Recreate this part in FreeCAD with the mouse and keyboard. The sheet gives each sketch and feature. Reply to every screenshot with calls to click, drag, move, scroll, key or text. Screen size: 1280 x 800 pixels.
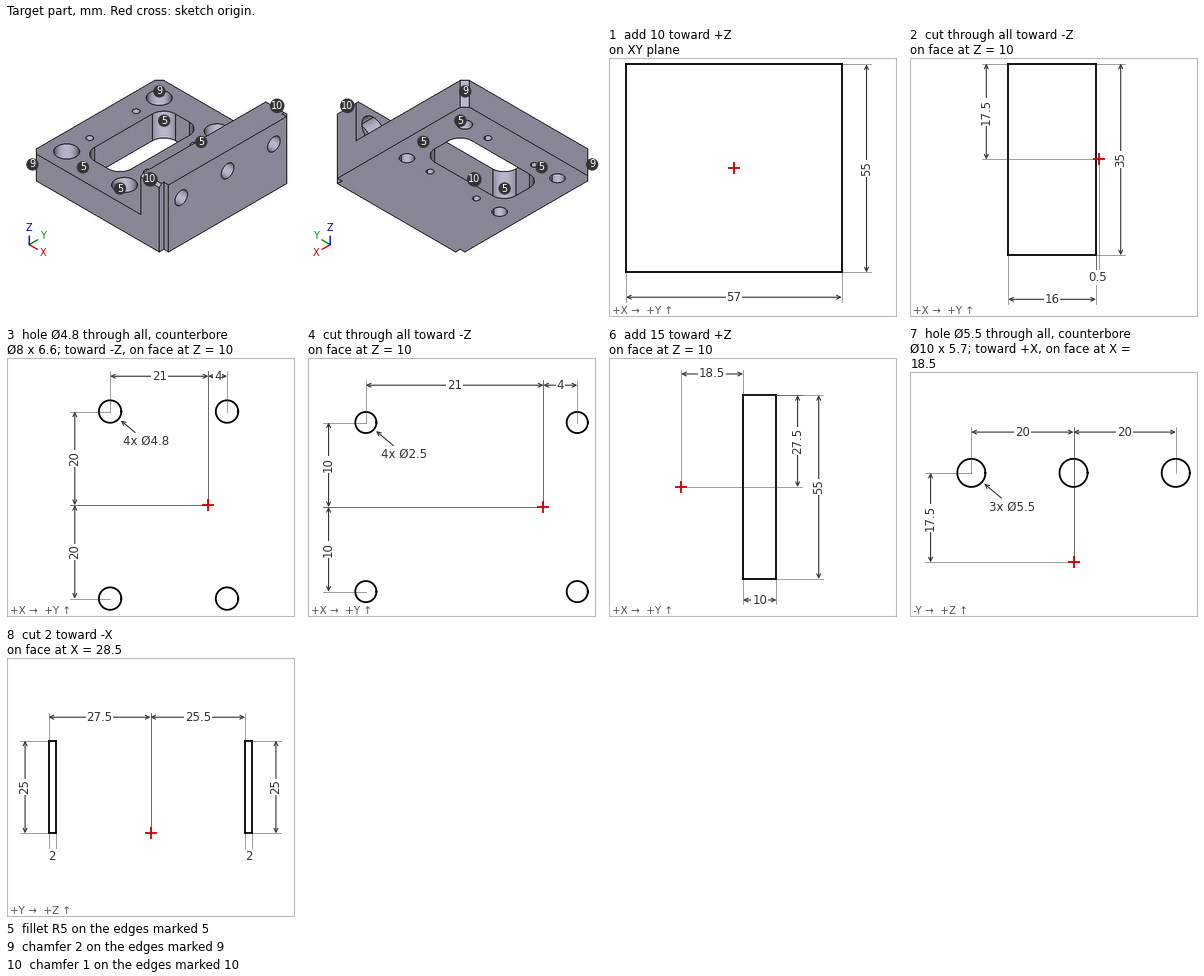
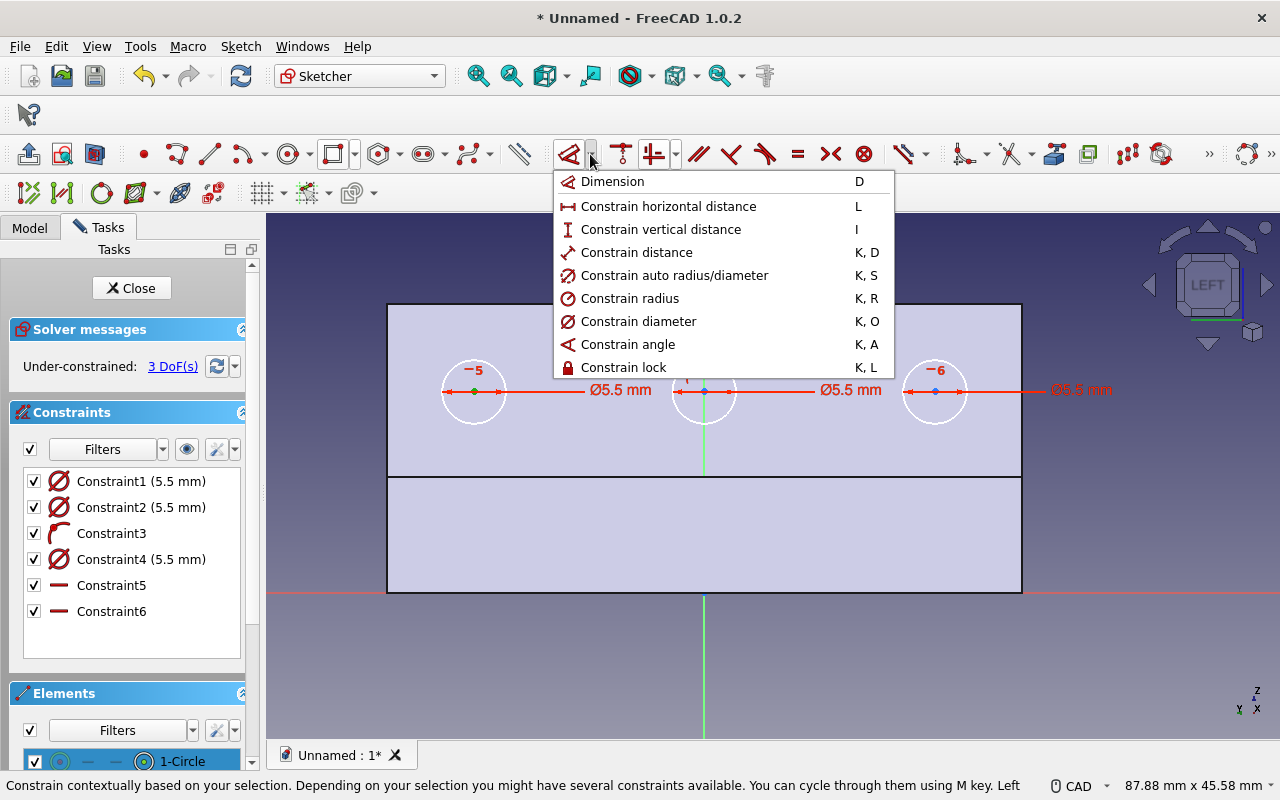
click(724, 206)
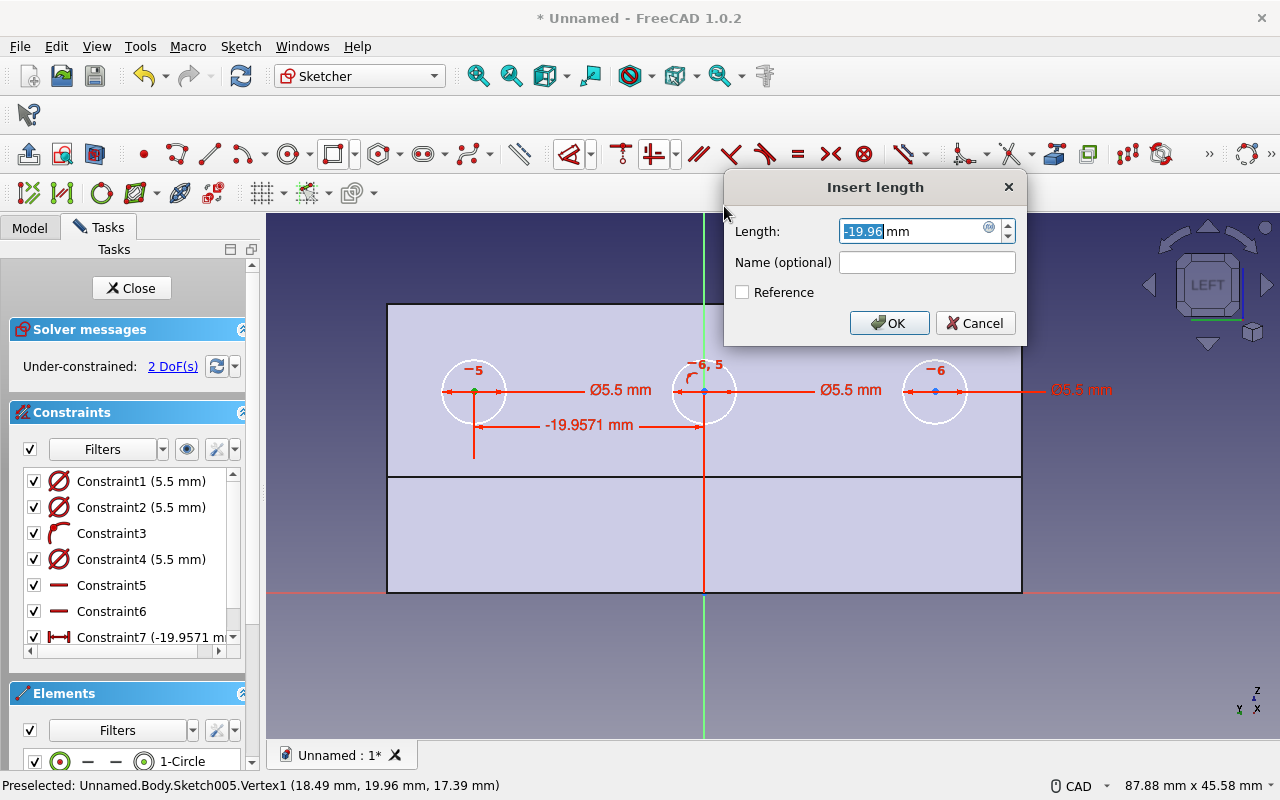
text(-20)
key(Return)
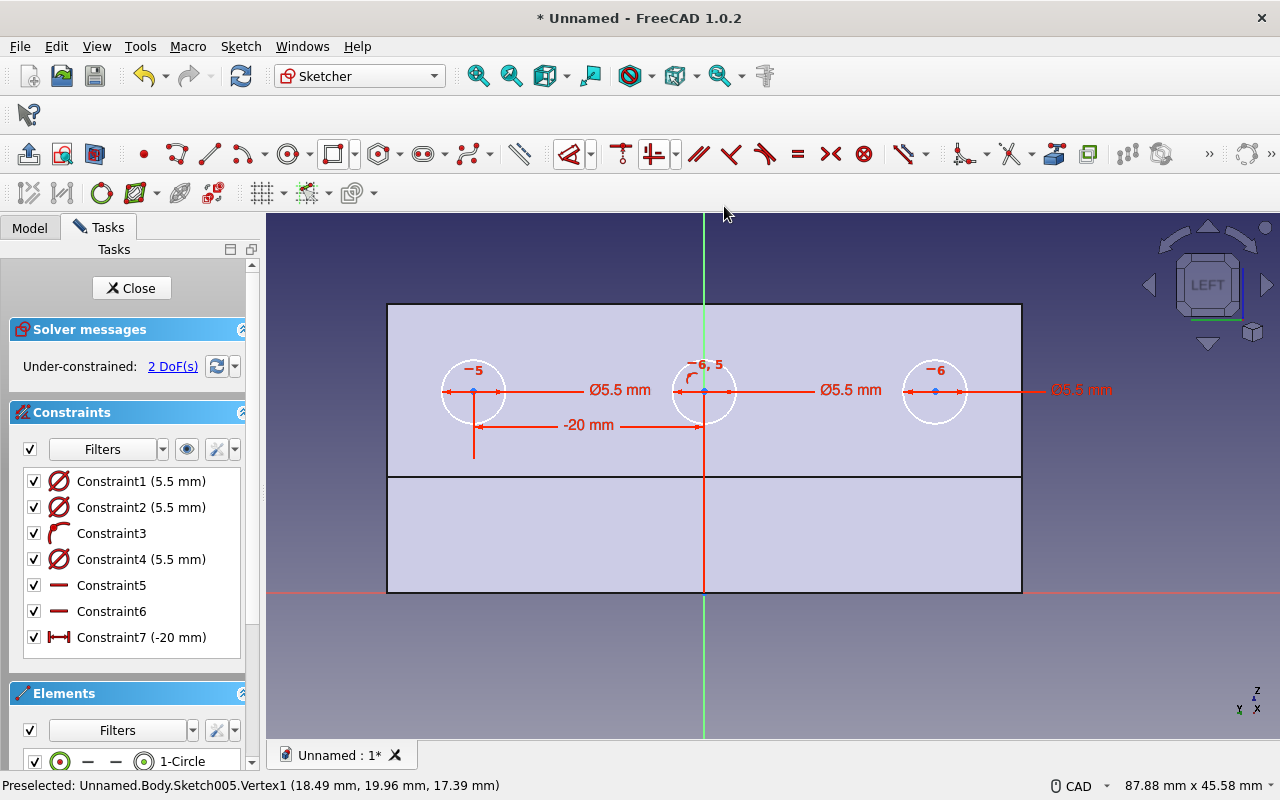
click(935, 392)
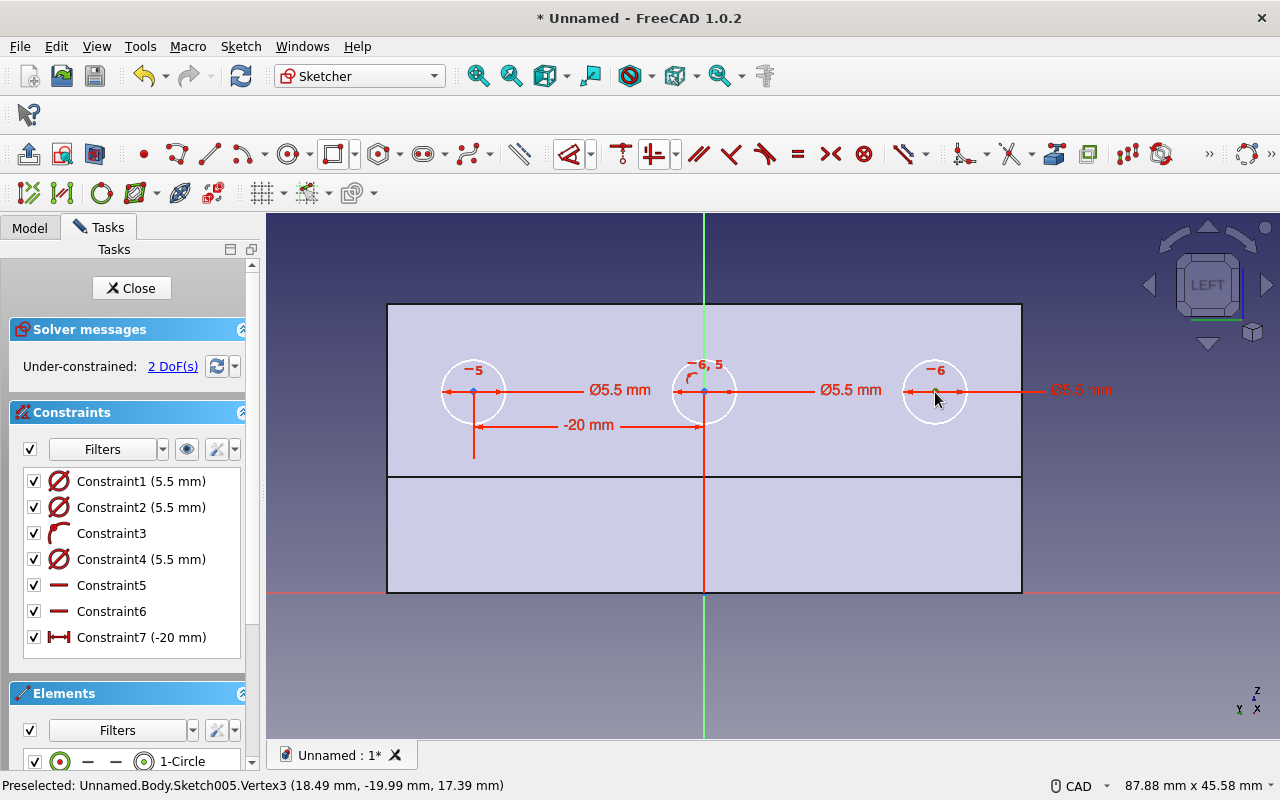
click(590, 154)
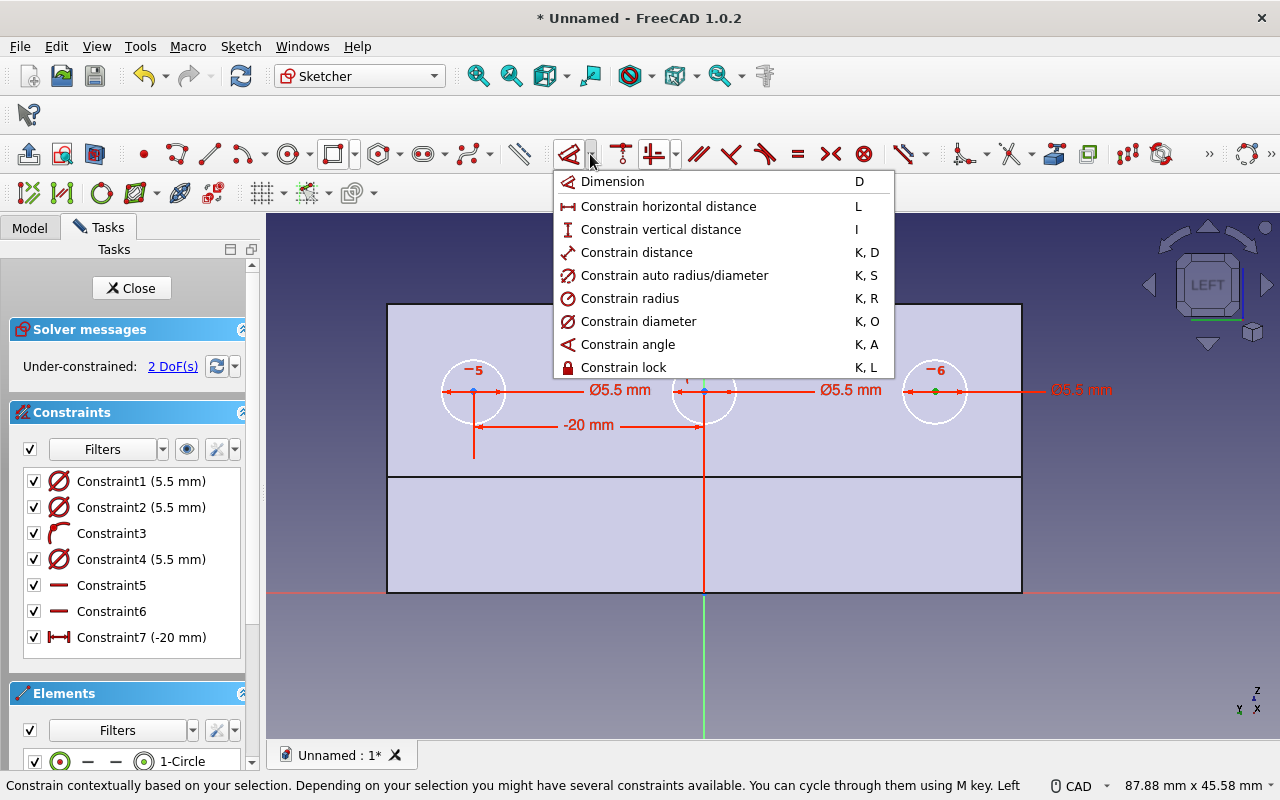
click(724, 206)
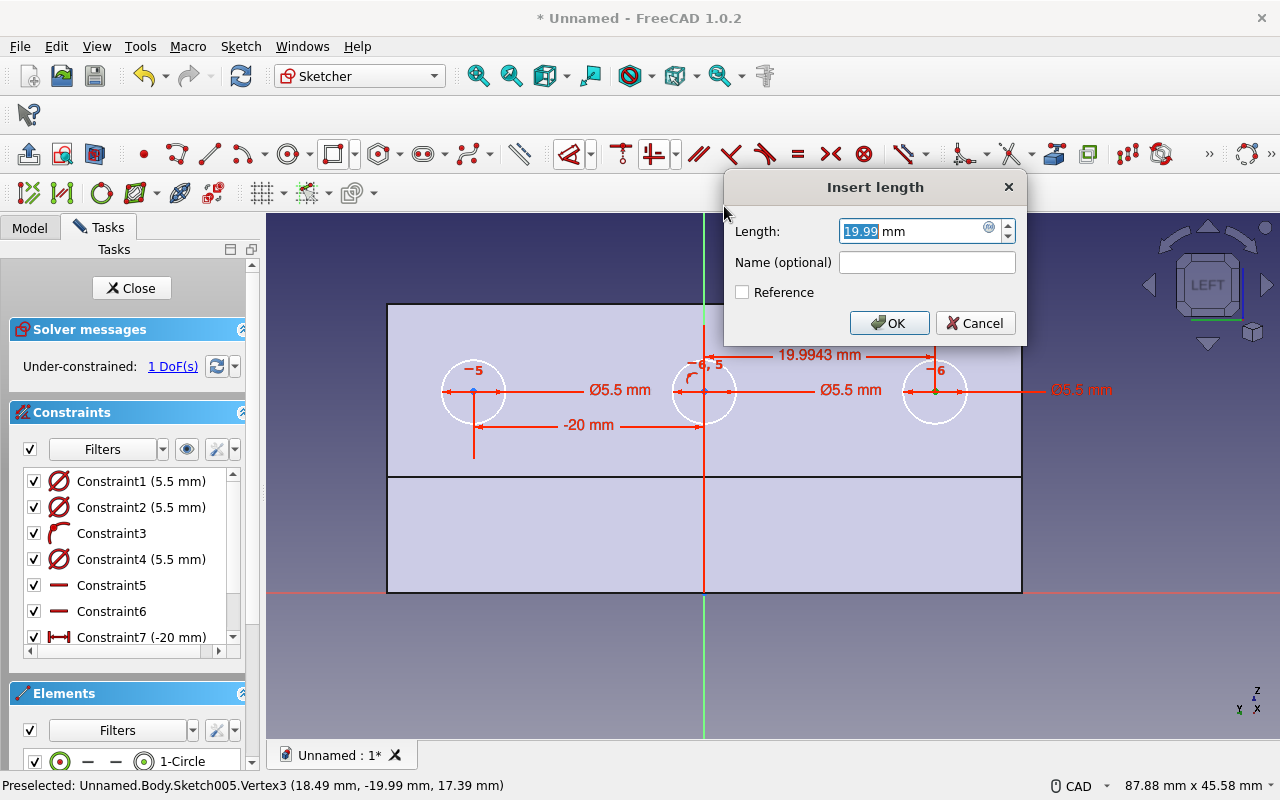
text(20)
key(Return)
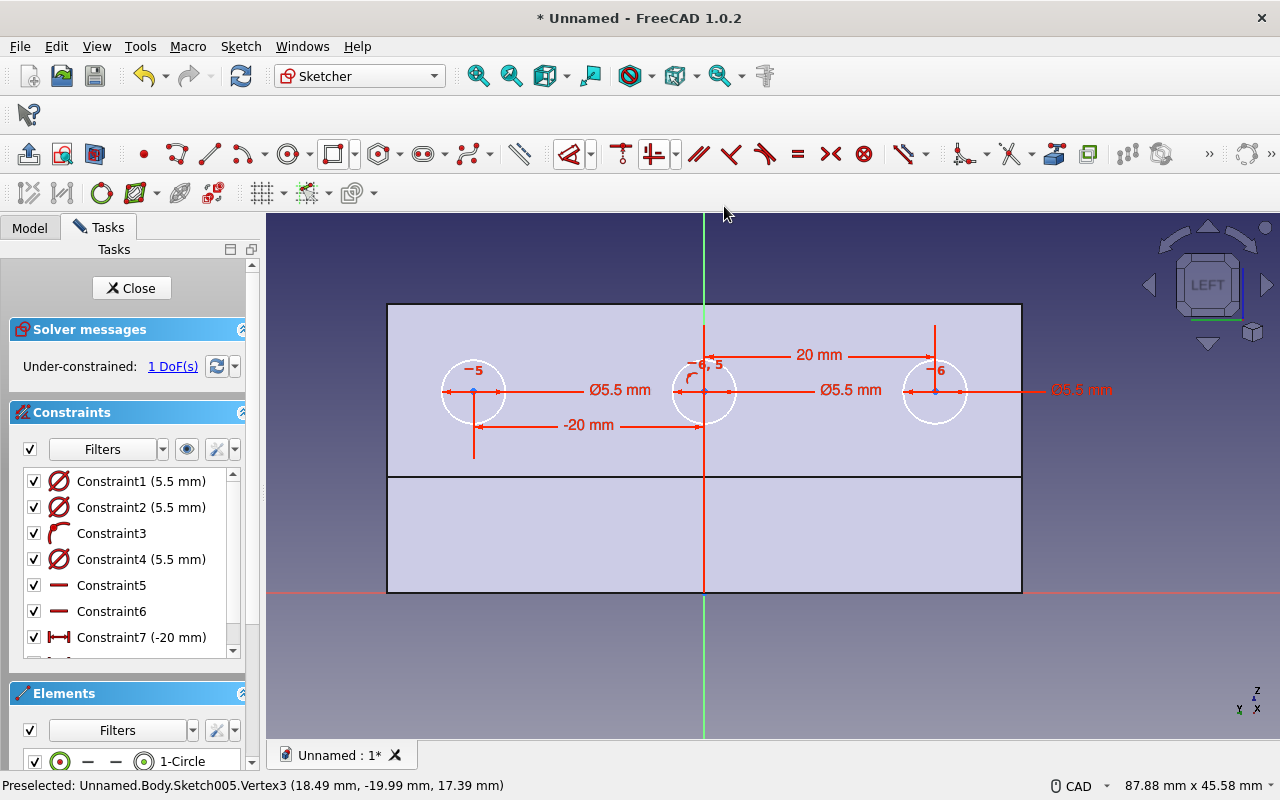
click(474, 392)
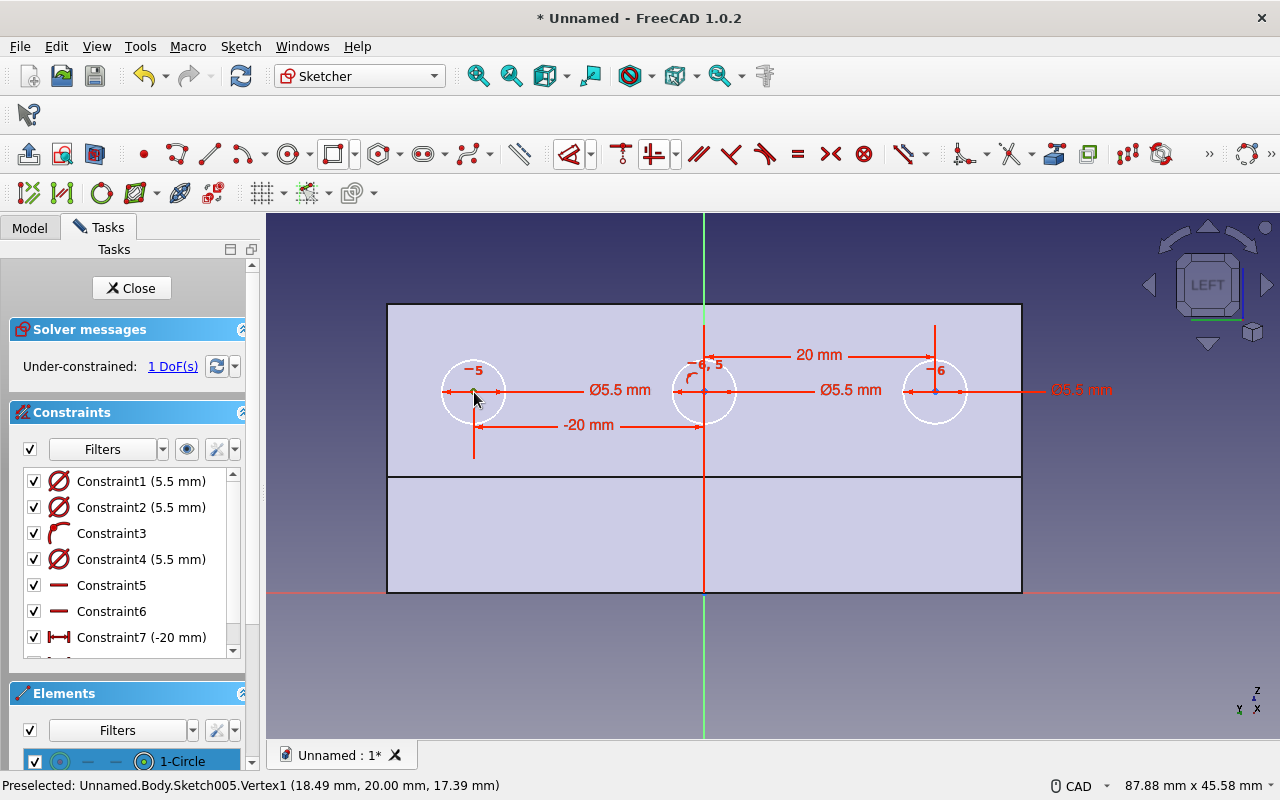
key(i)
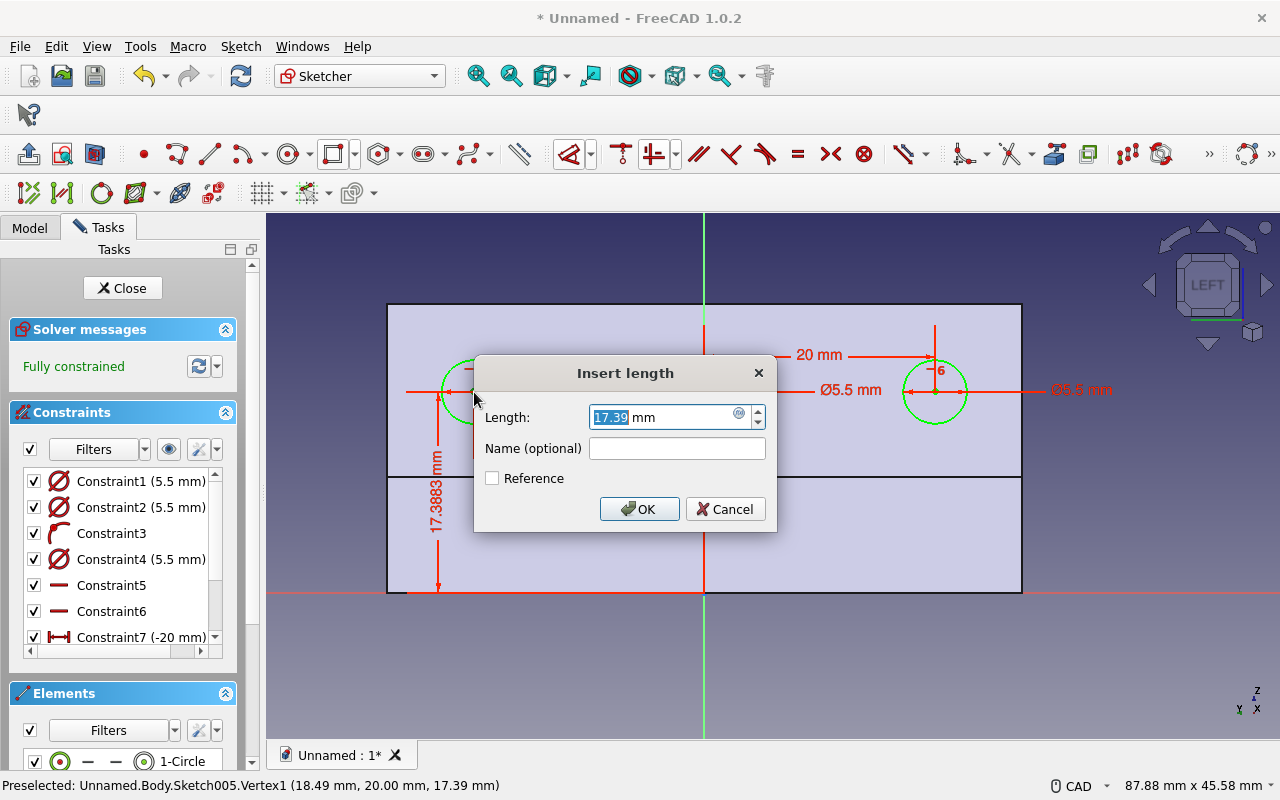
text(17.5)
key(Return)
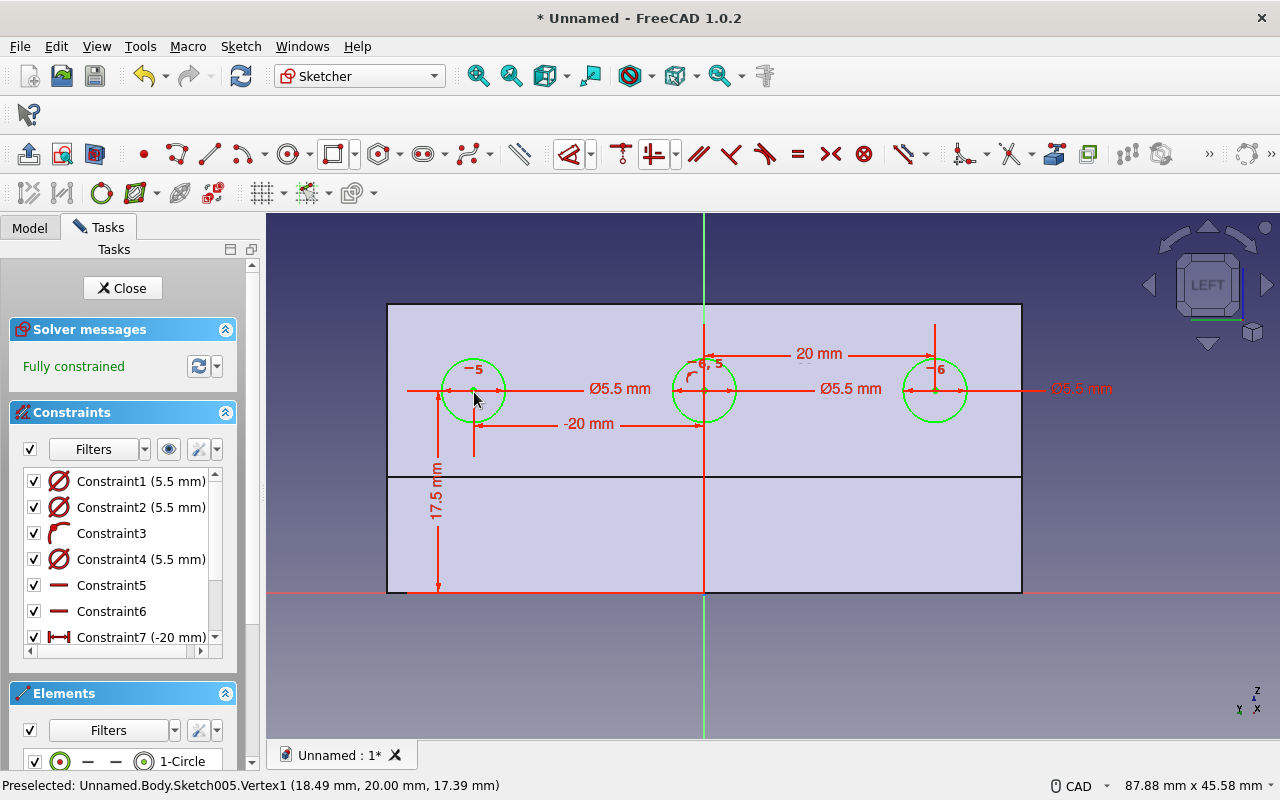
click(123, 288)